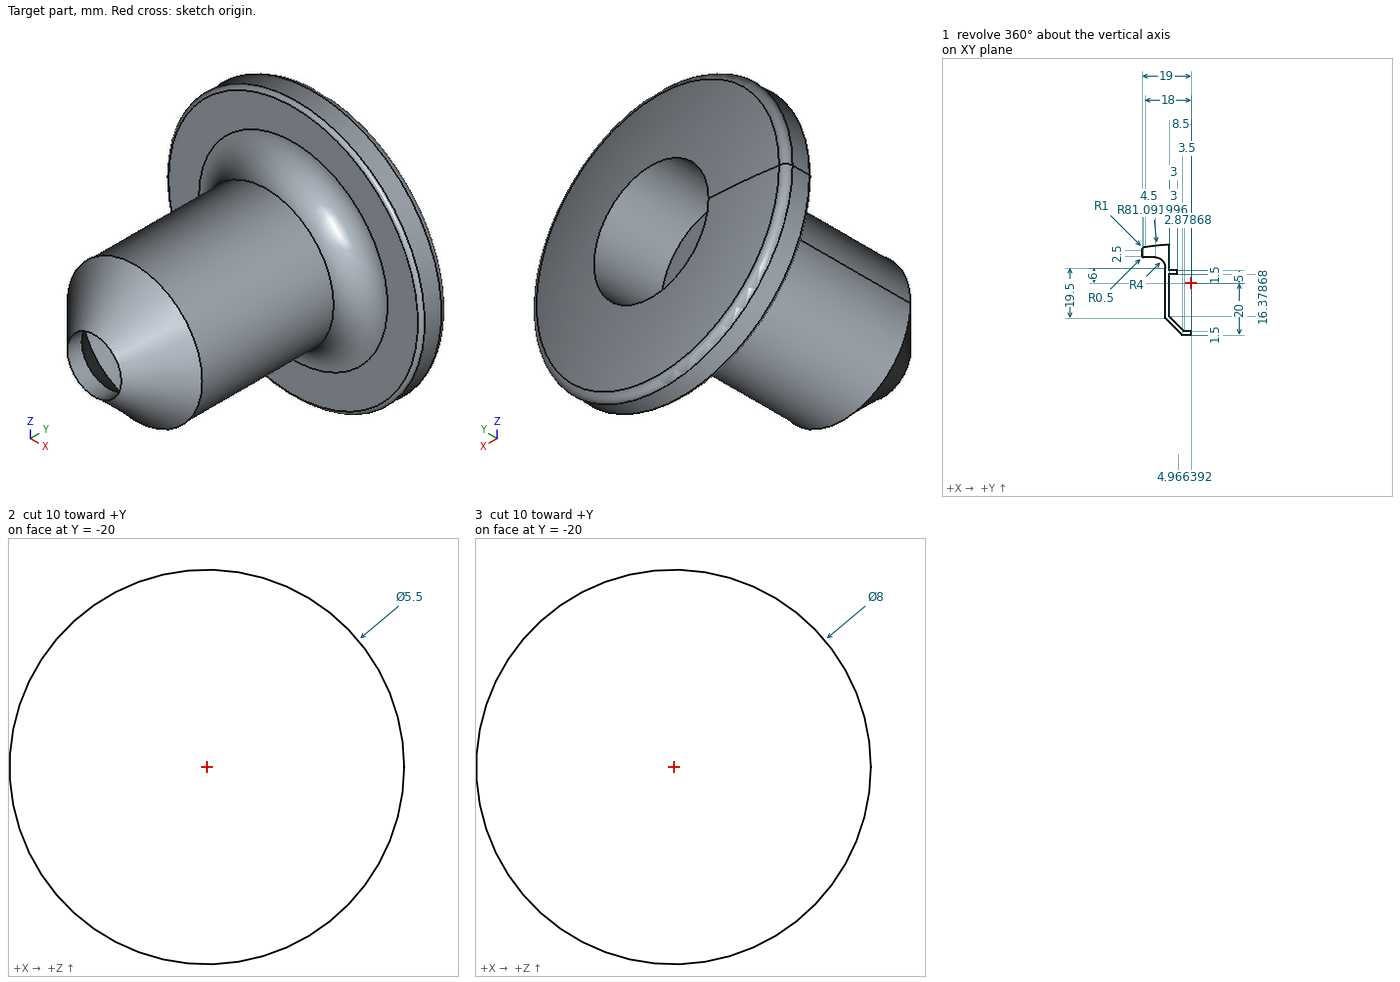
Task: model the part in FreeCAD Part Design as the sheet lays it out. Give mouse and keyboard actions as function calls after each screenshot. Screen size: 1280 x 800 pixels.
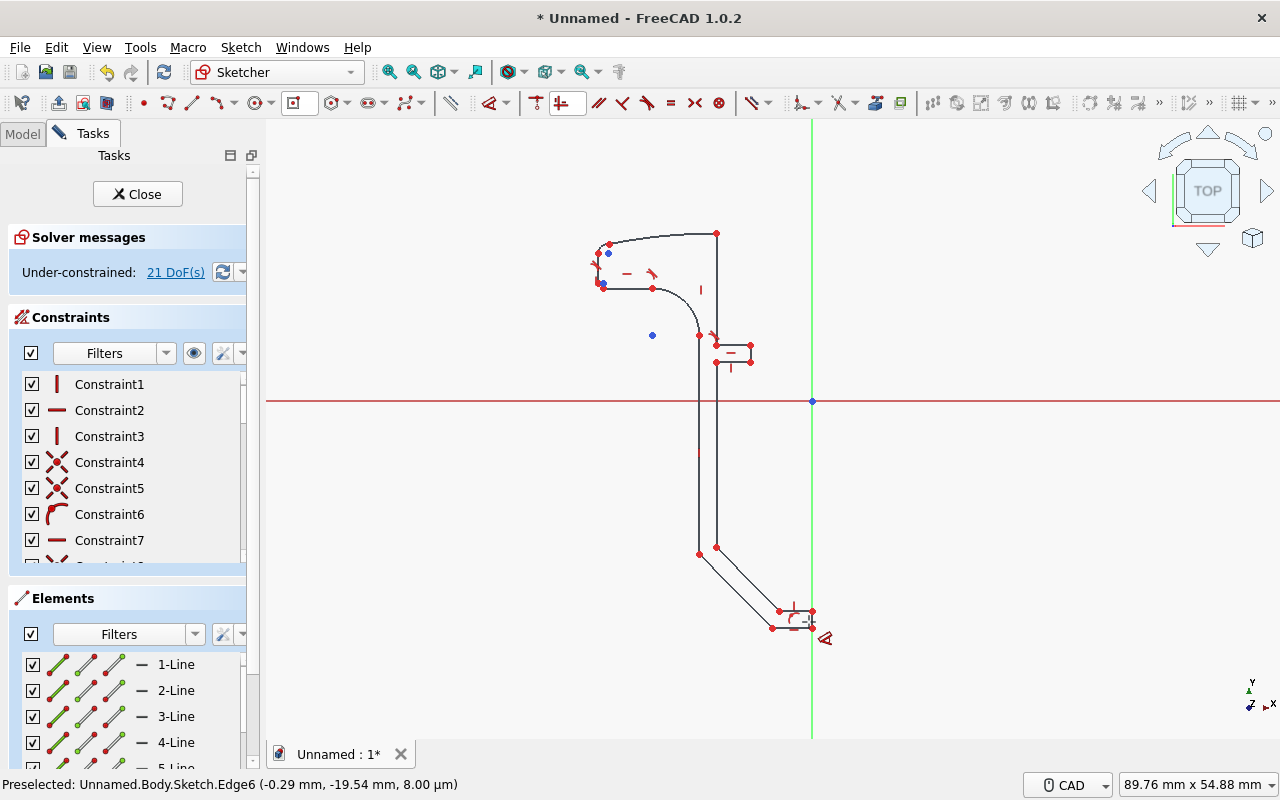
scroll(600, 287, up, 10)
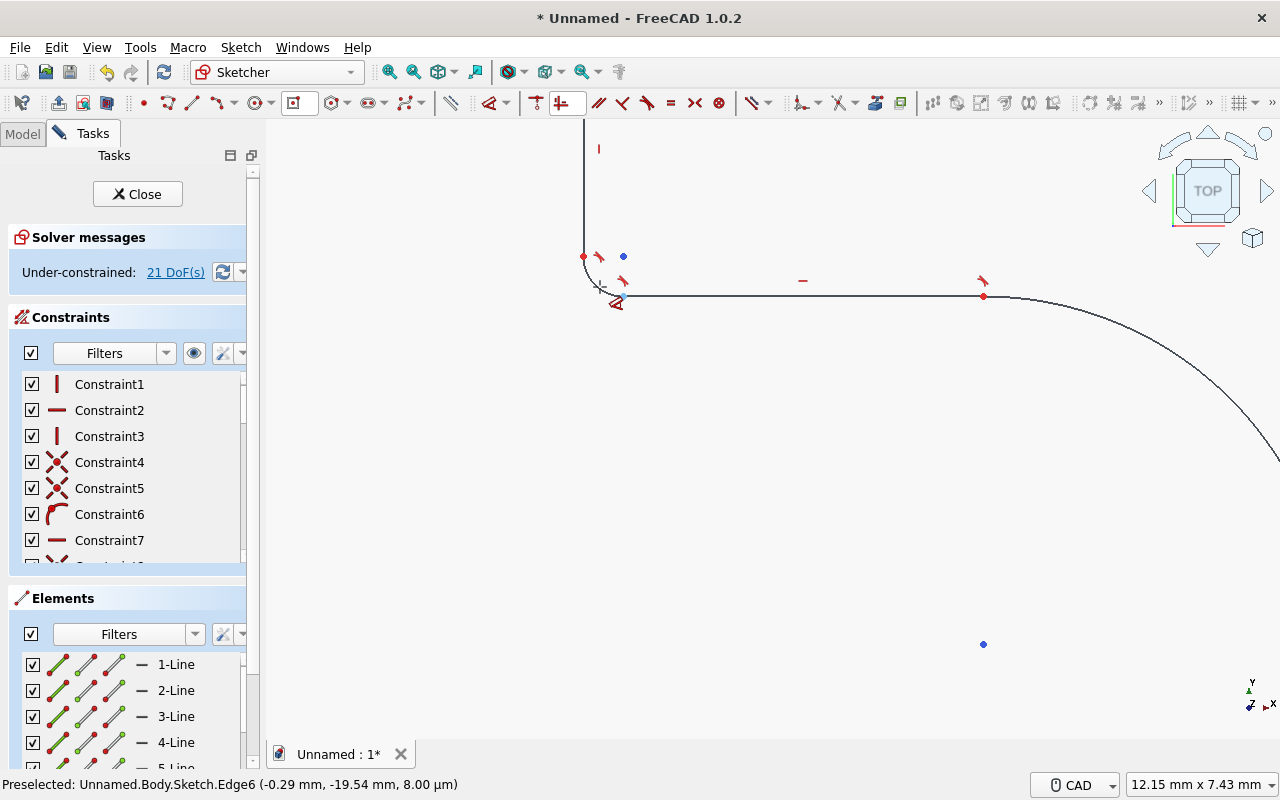
click(595, 285)
click(572, 308)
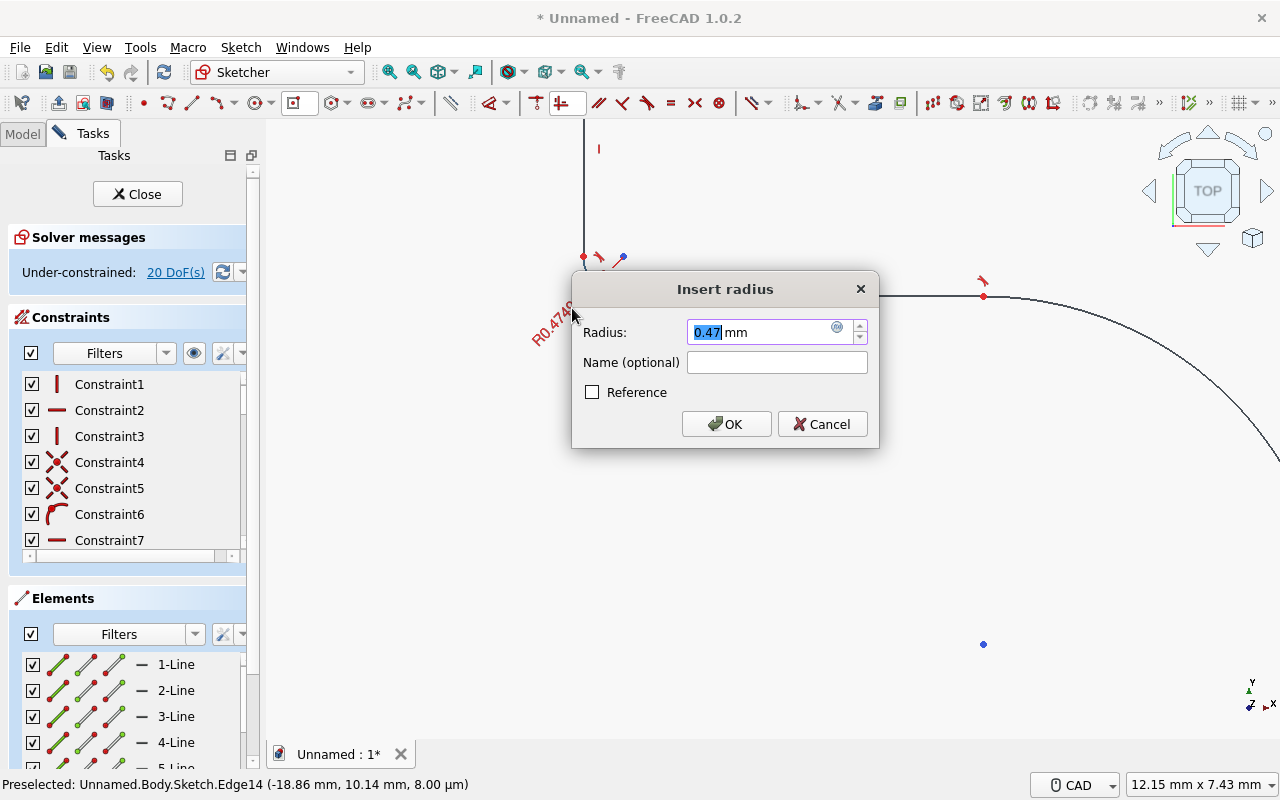
text(0.5)
key(Return)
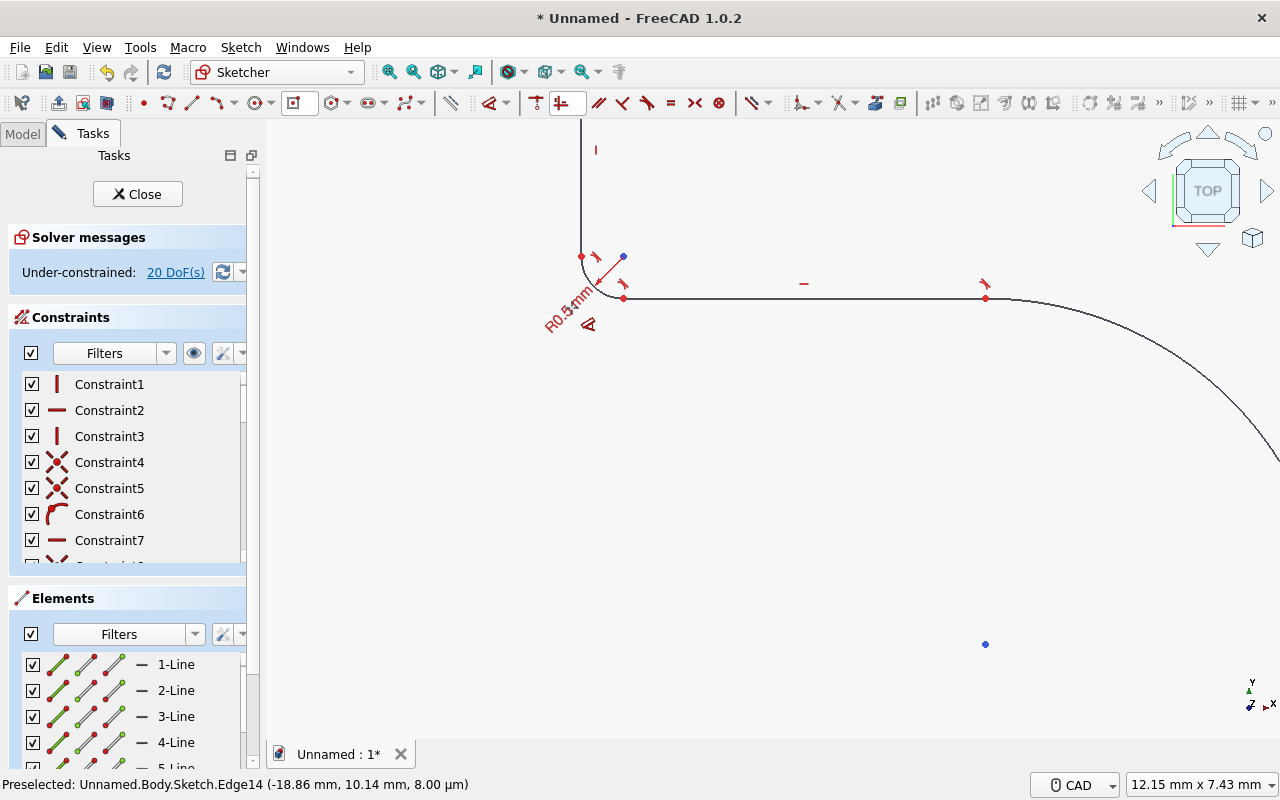
scroll(600, 287, down, 10)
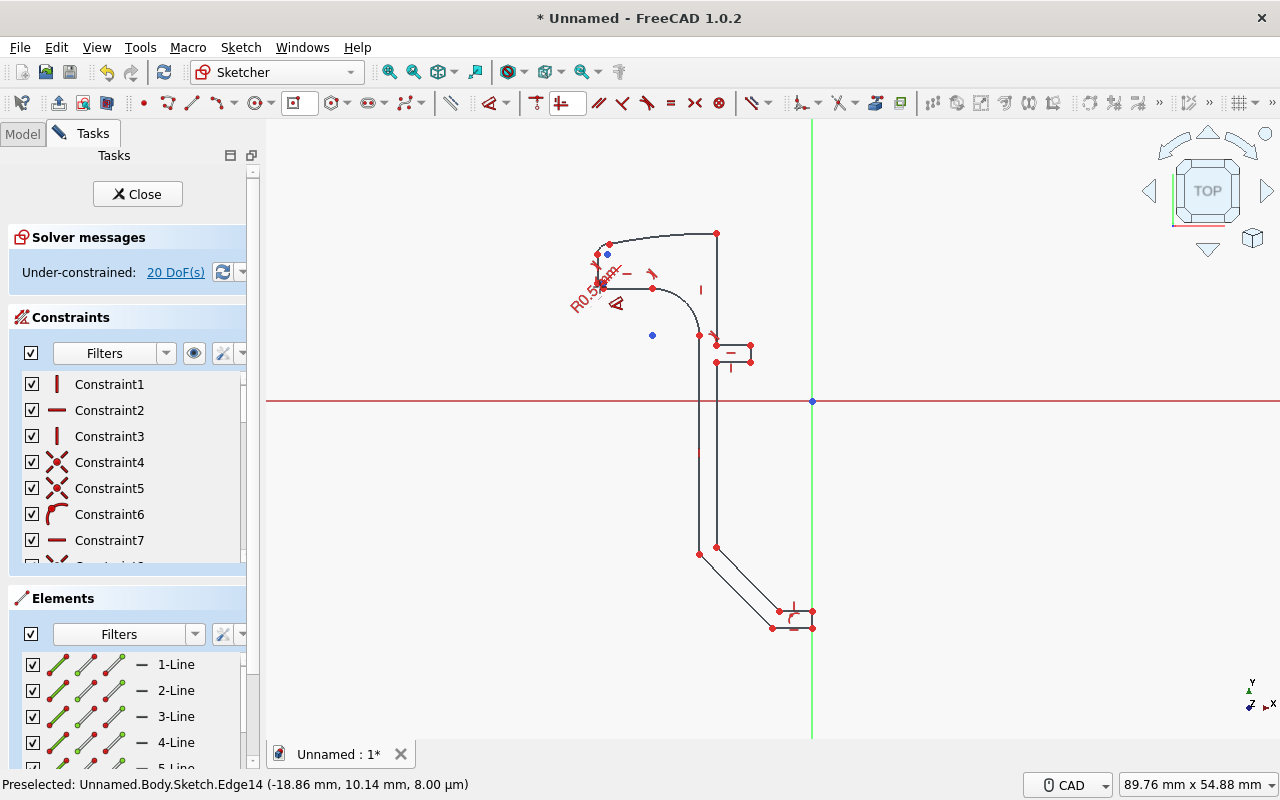
click(667, 291)
click(677, 261)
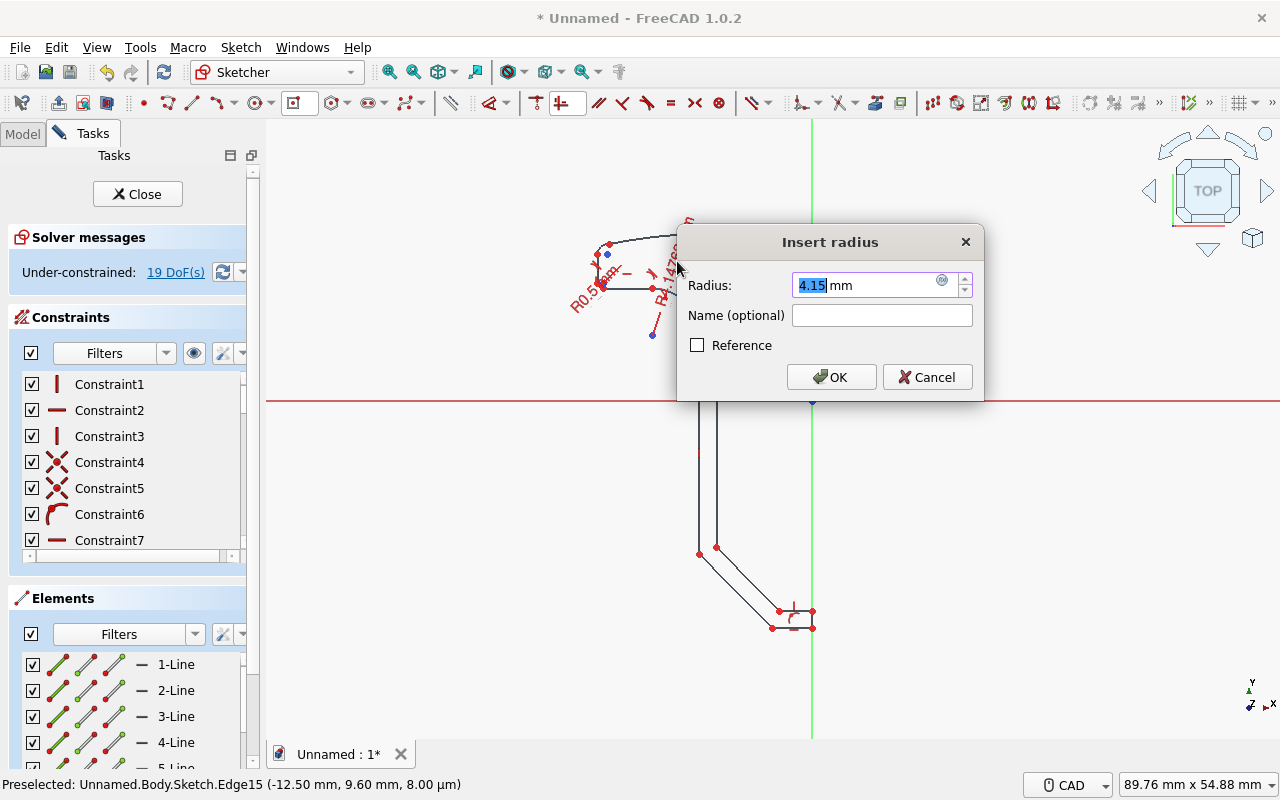
text(4)
key(Return)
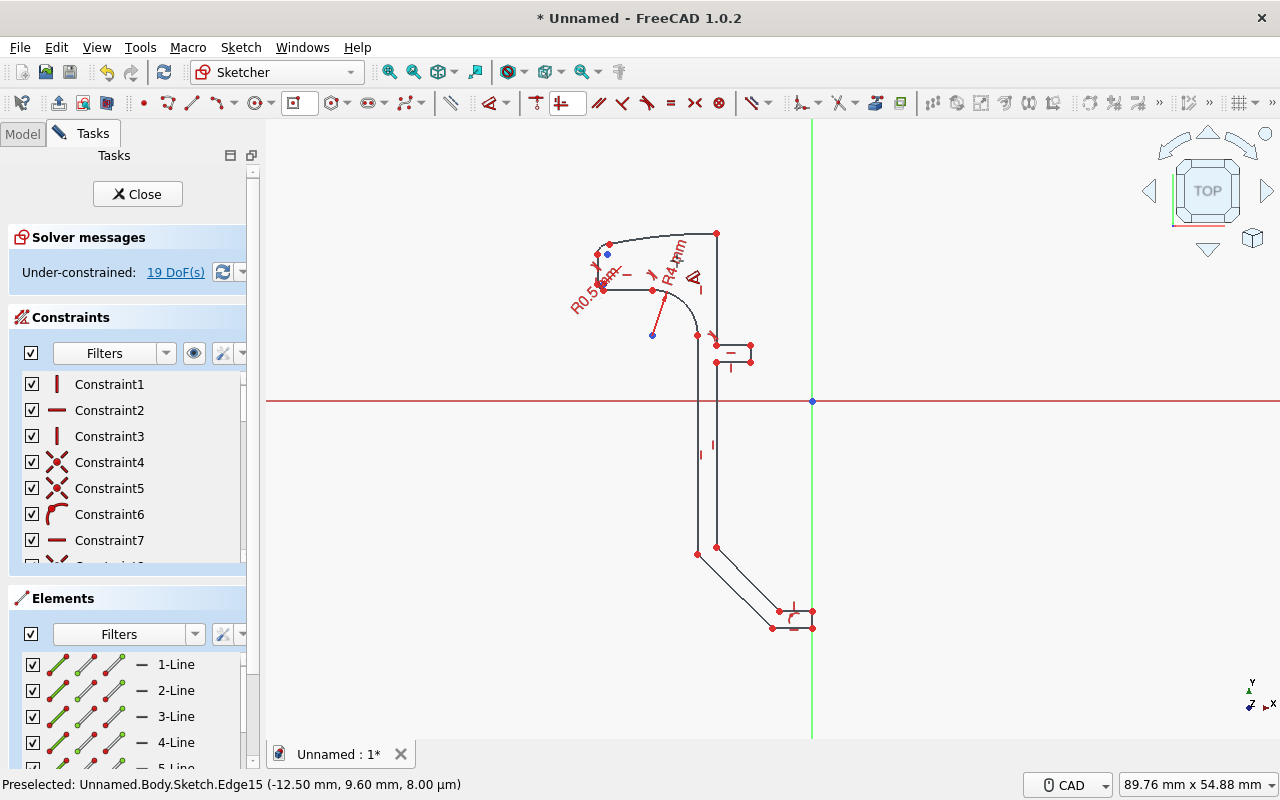
click(684, 234)
click(682, 202)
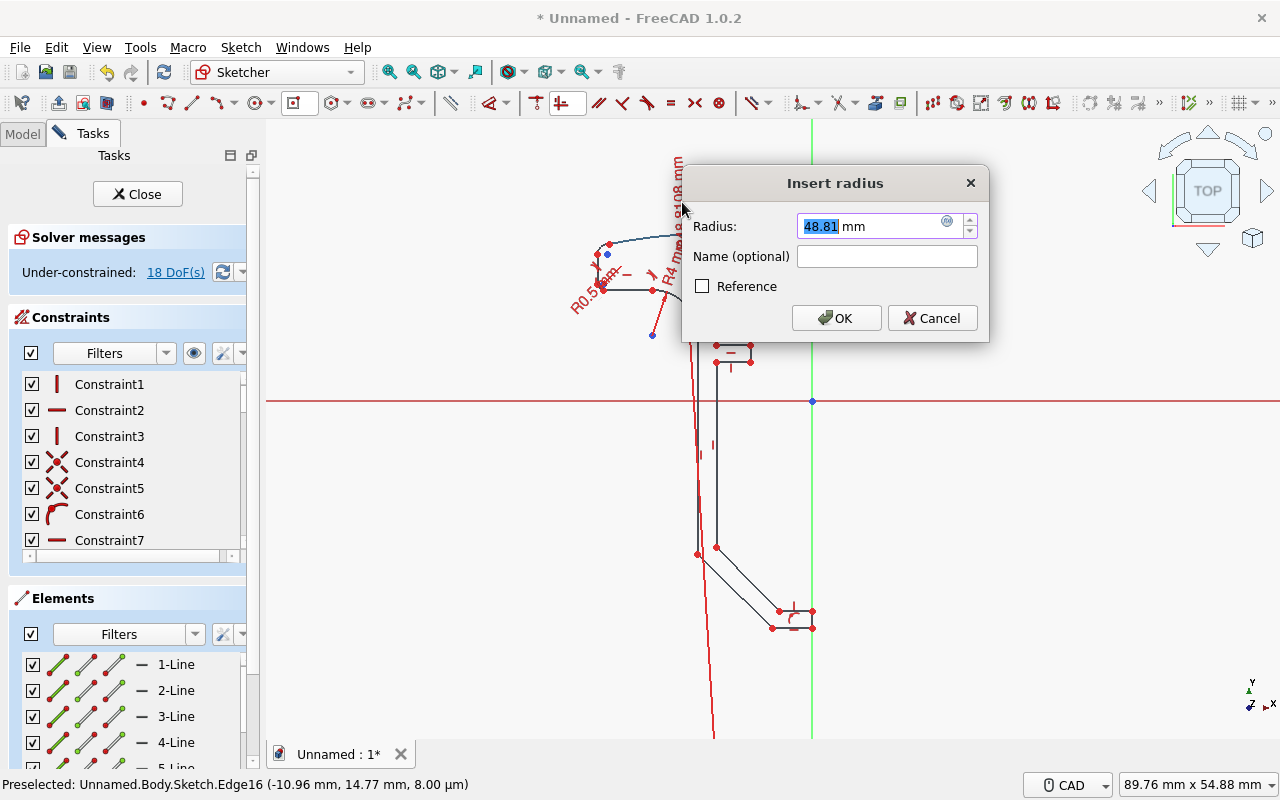
text(81.091996)
key(Return)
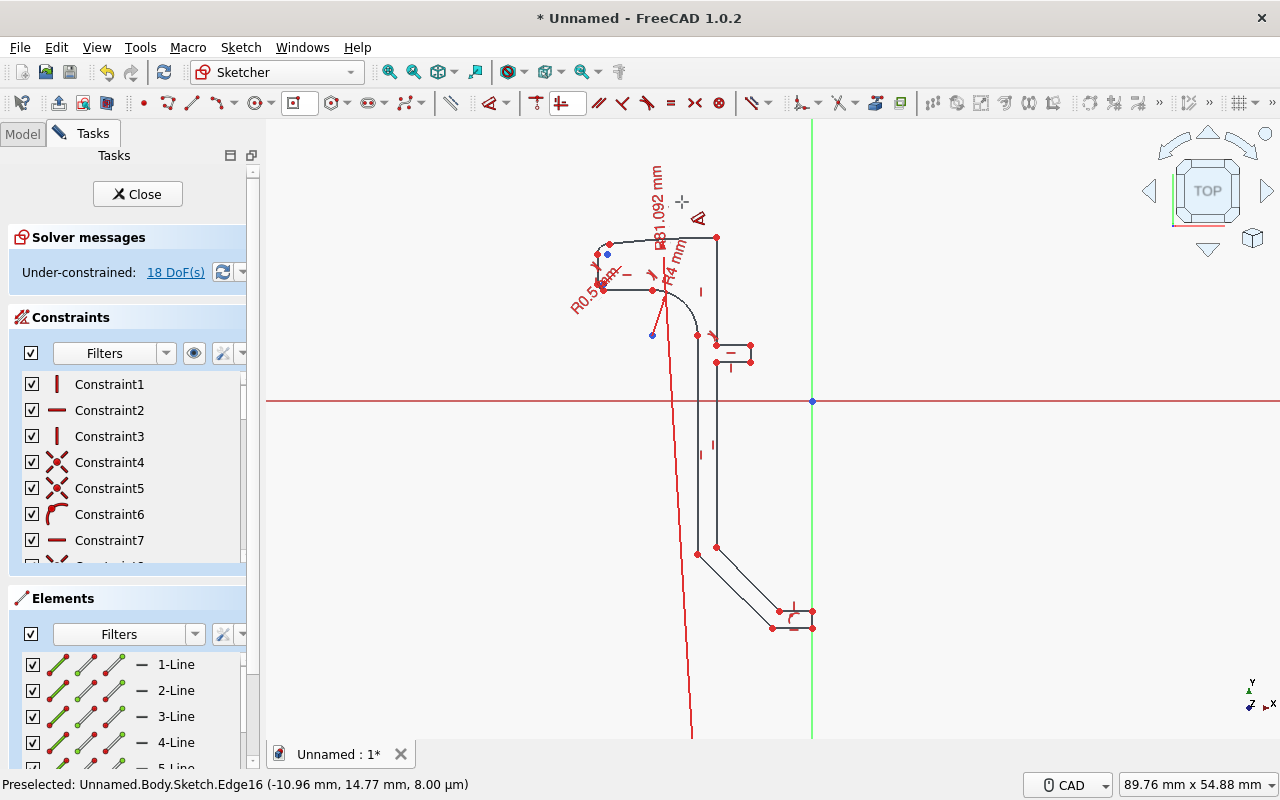
scroll(601, 247, up, 7)